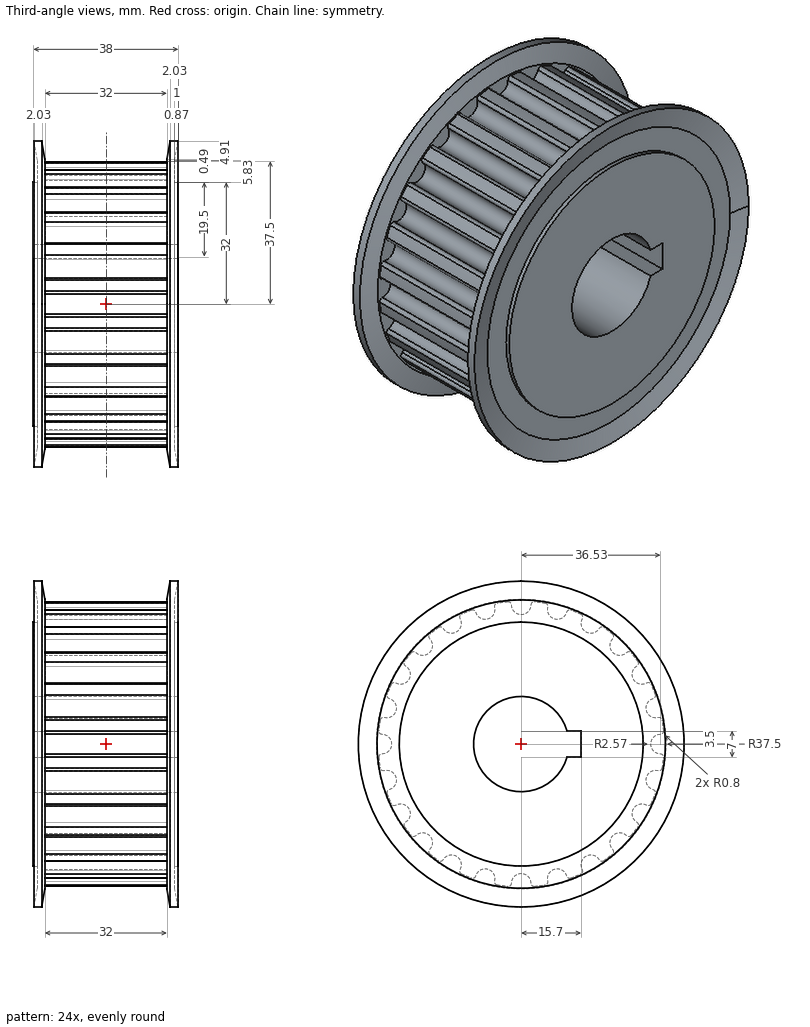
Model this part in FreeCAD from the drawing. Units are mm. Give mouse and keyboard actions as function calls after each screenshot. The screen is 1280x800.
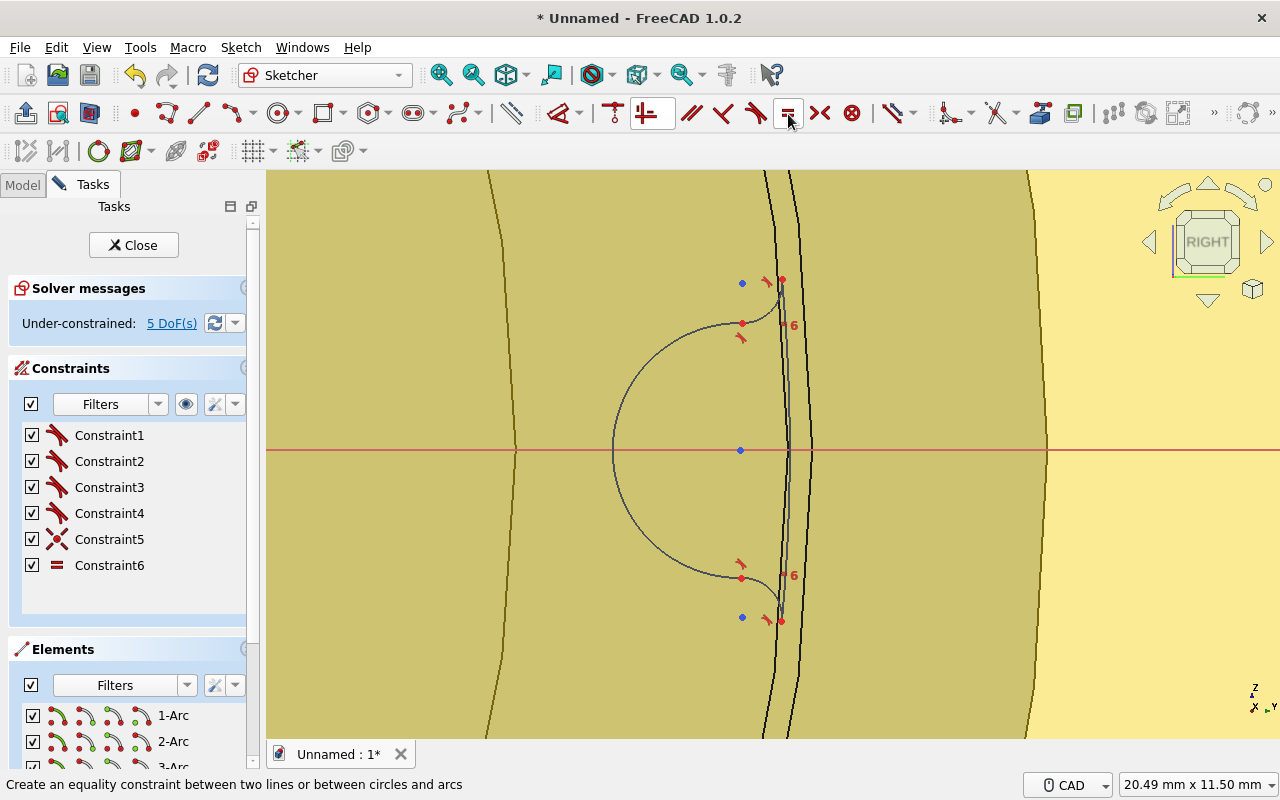
click(740, 451)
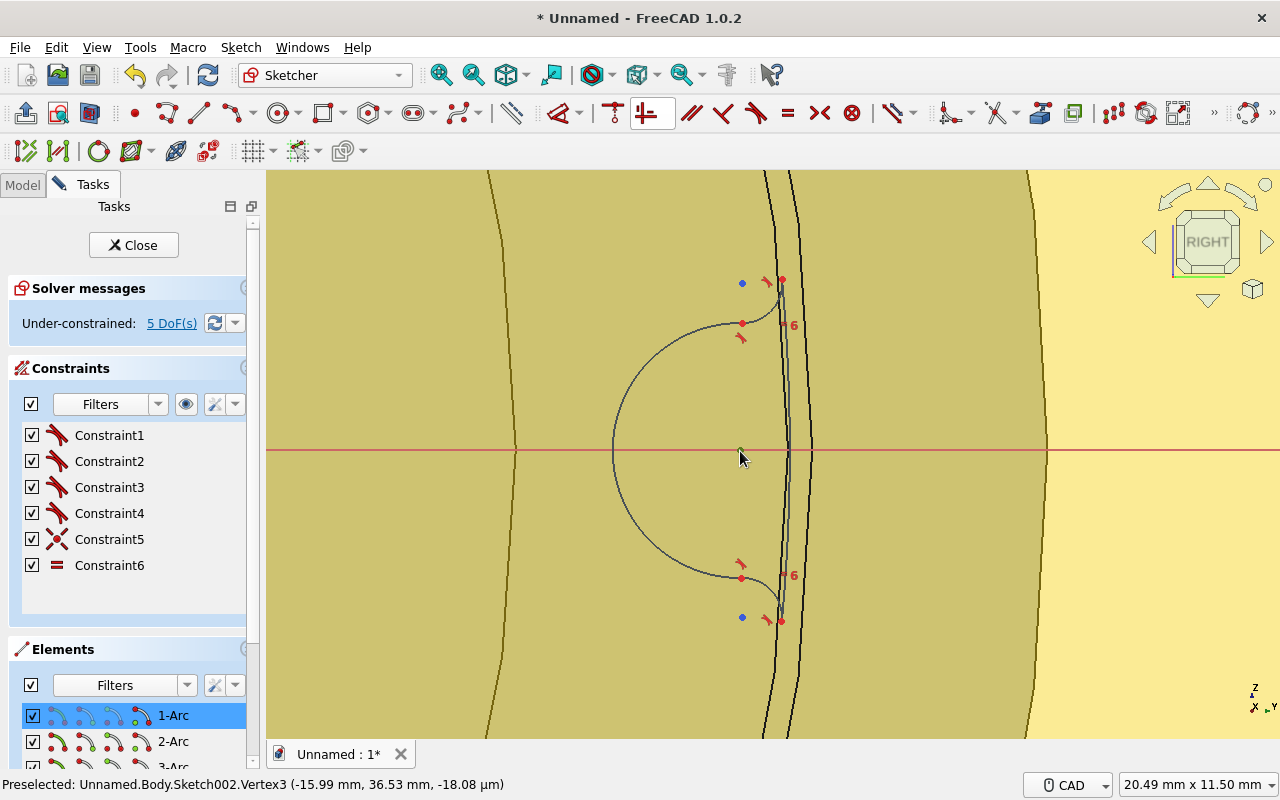
click(353, 450)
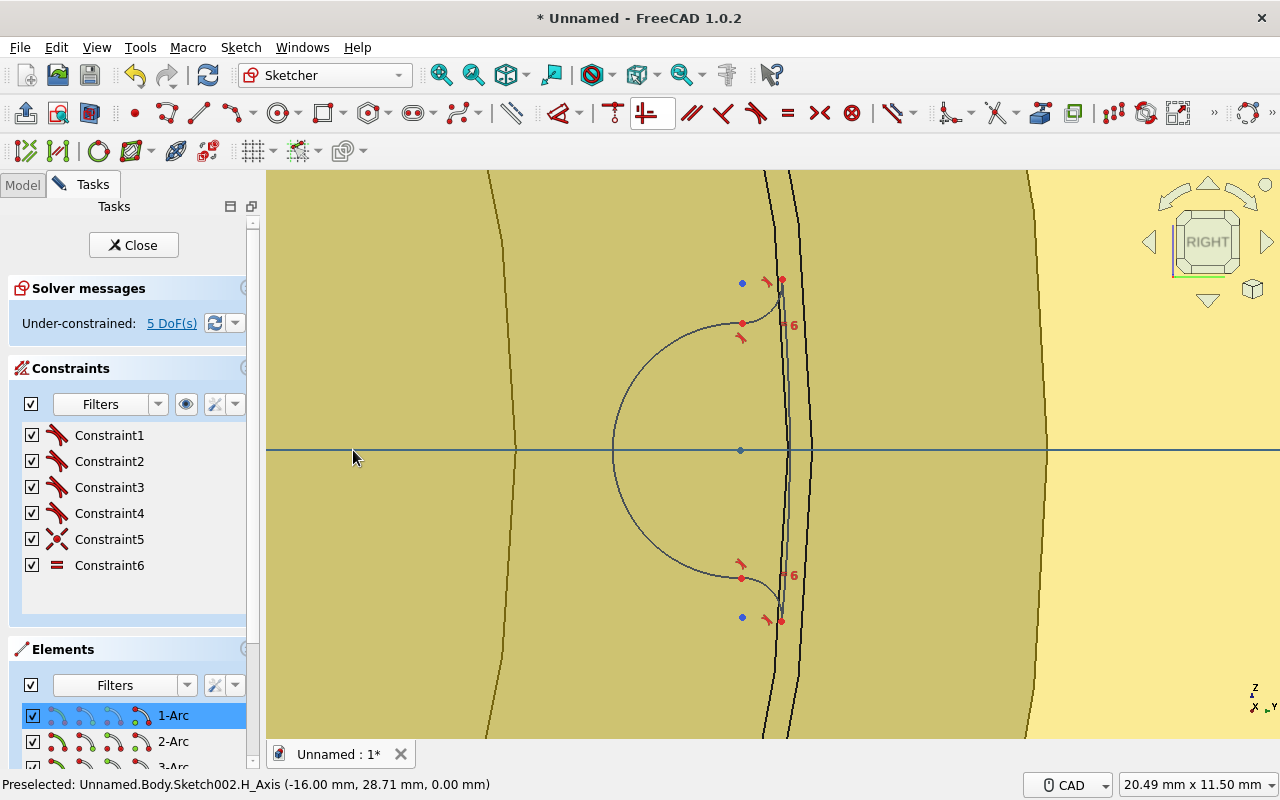
click(614, 114)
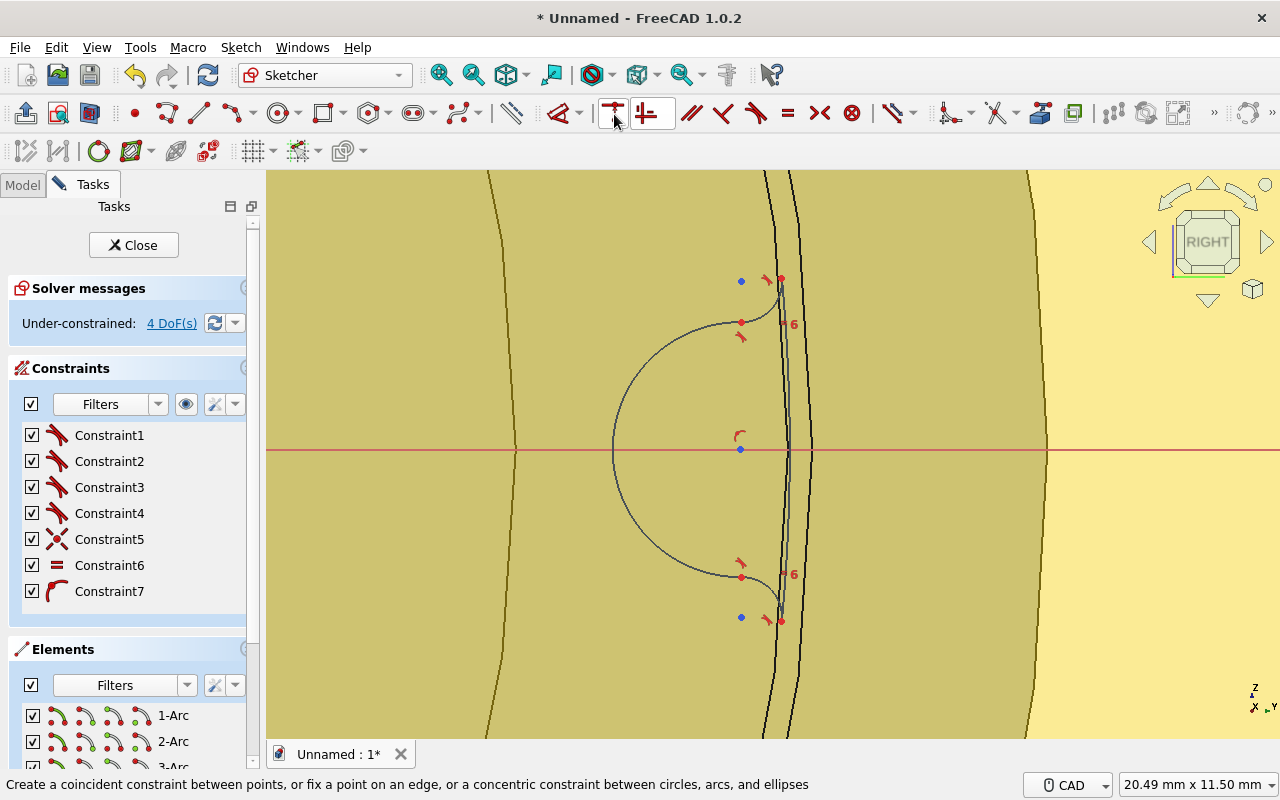
click(558, 114)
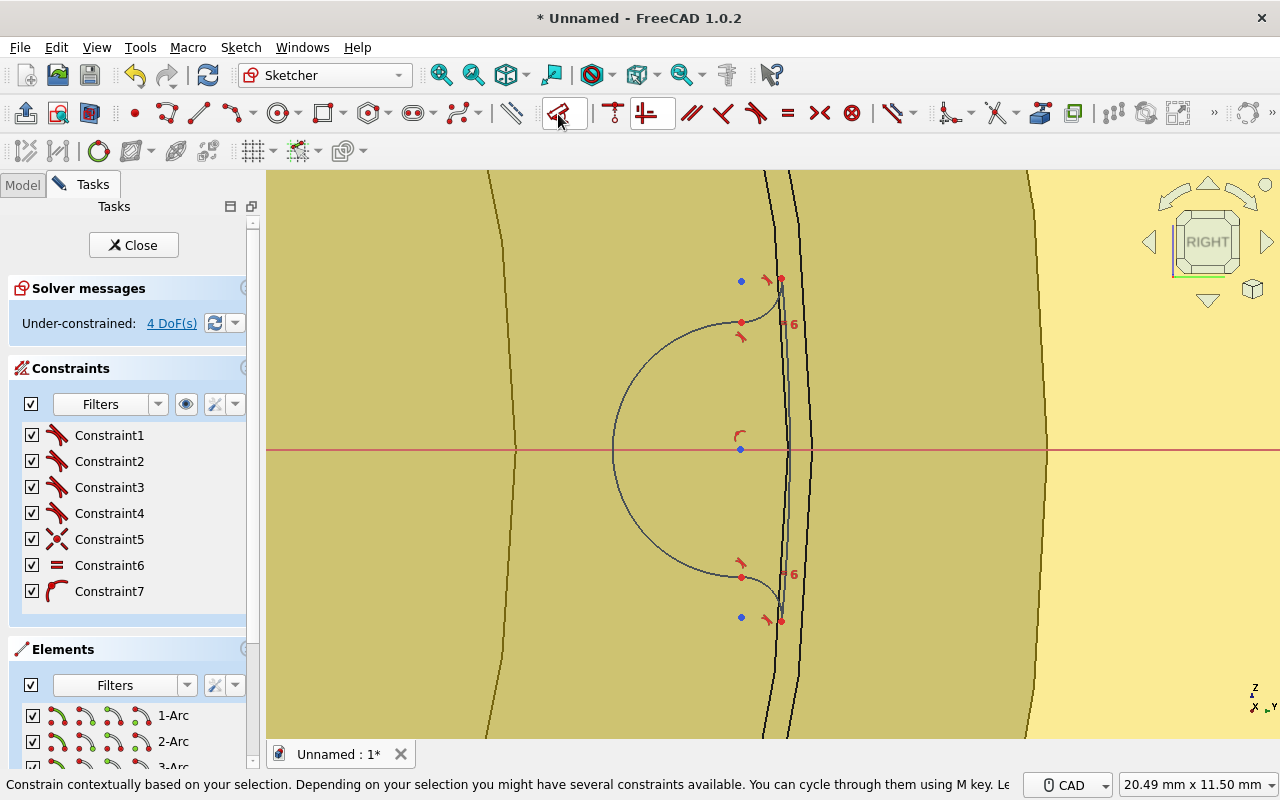
click(637, 374)
click(611, 355)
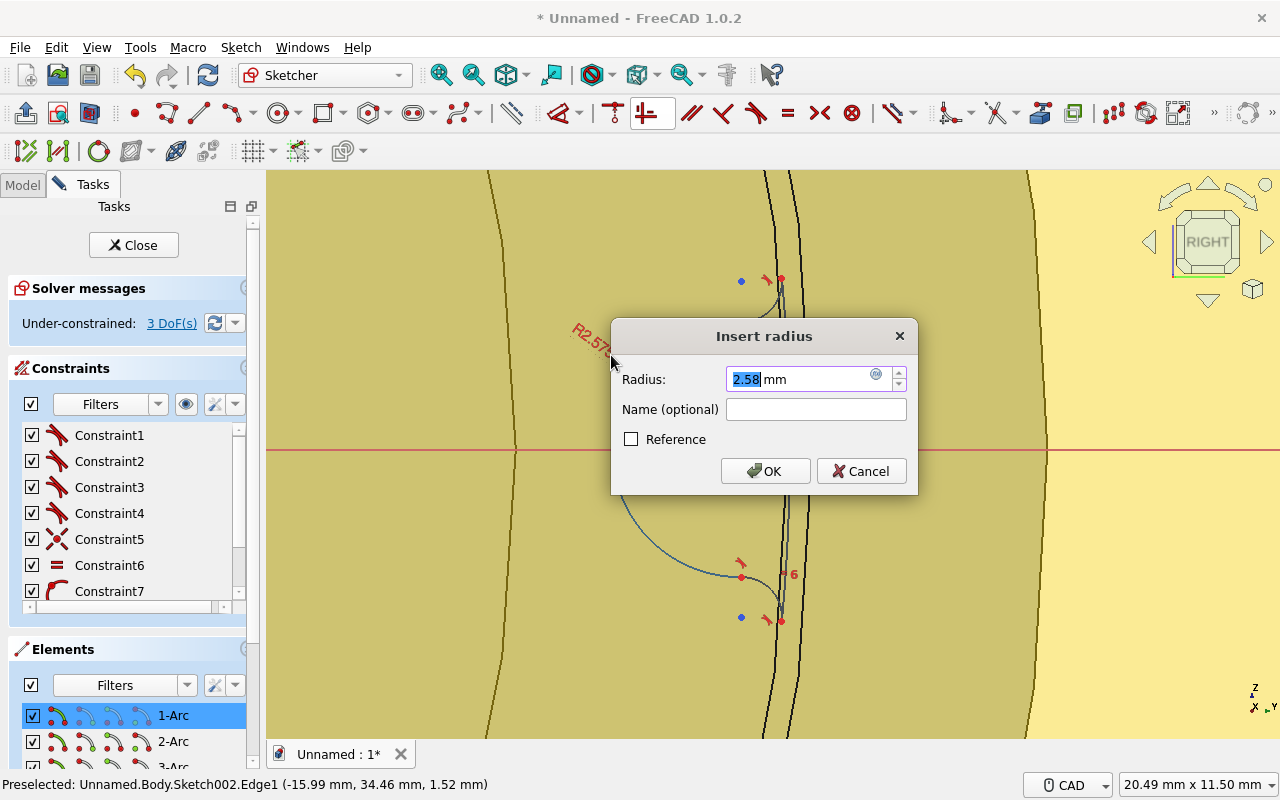
text(2.57)
key(Return)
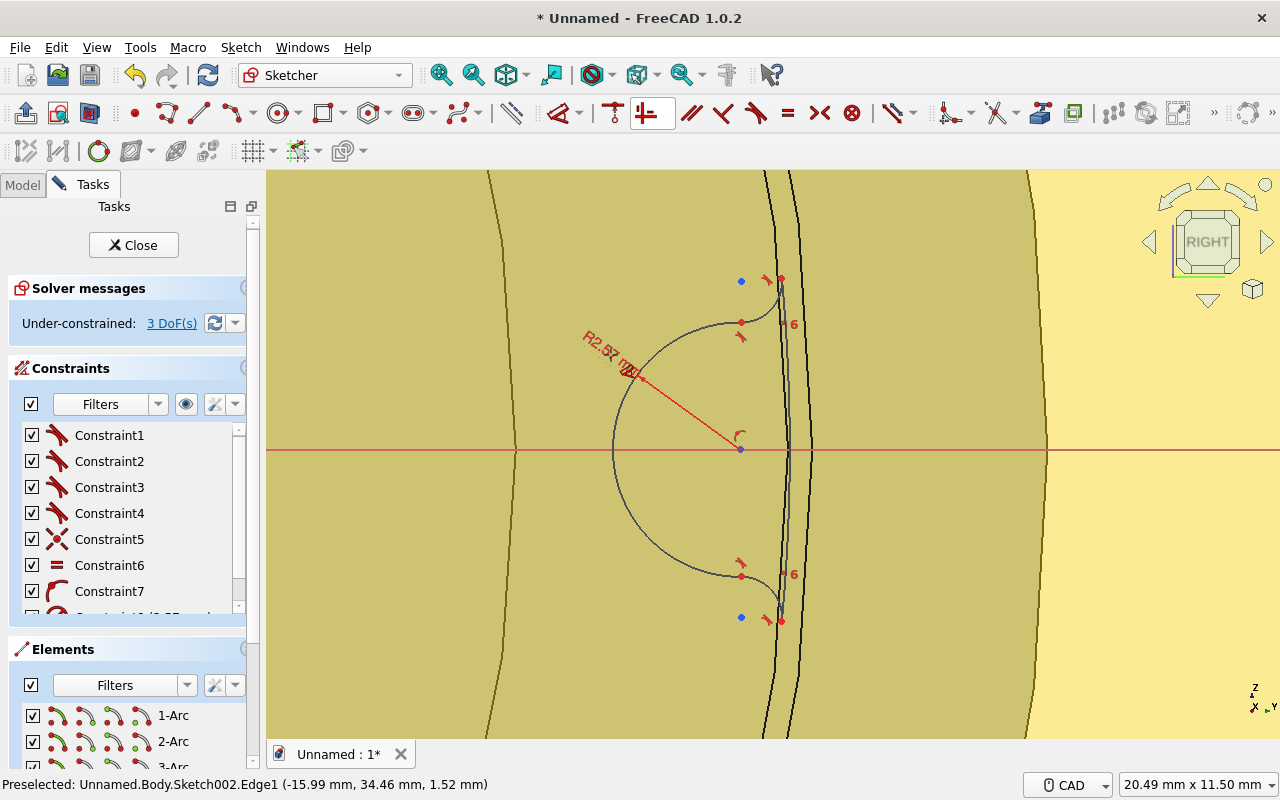
click(761, 582)
click(803, 579)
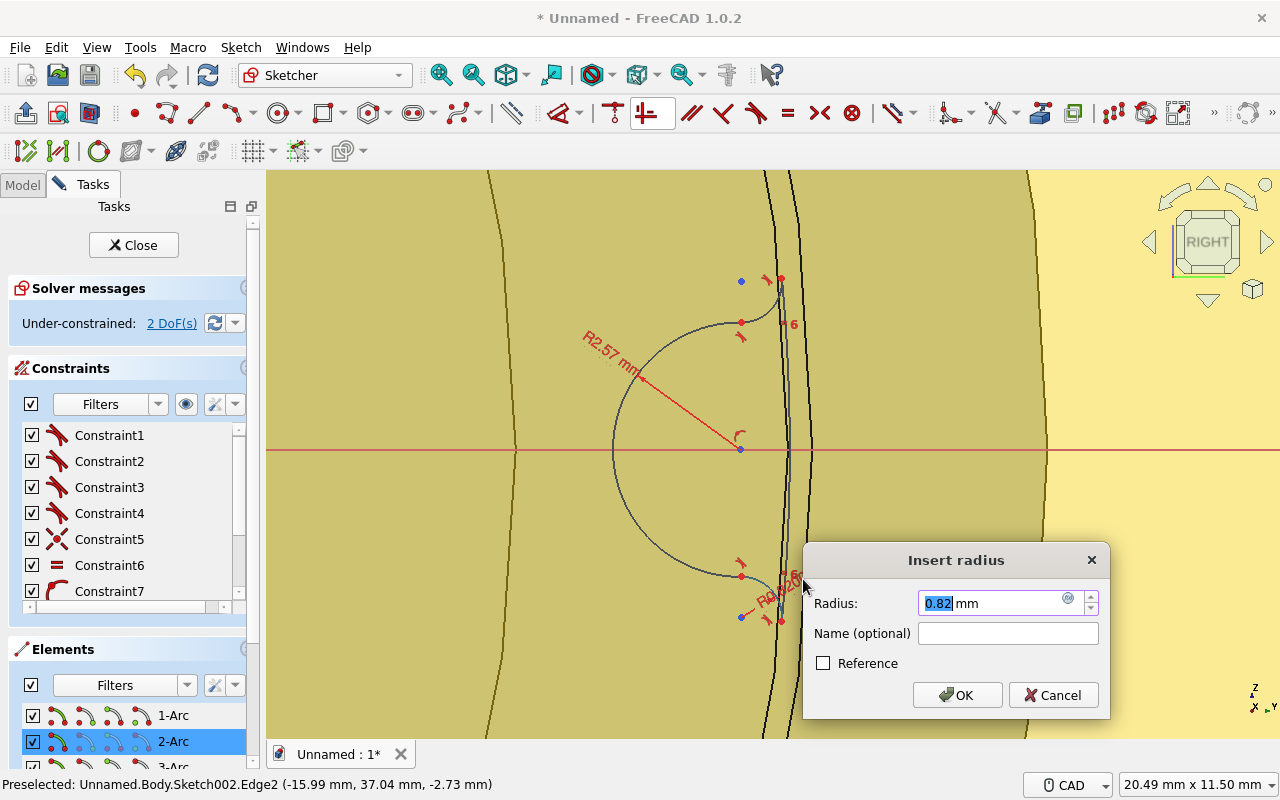
text(0.8)
key(Return)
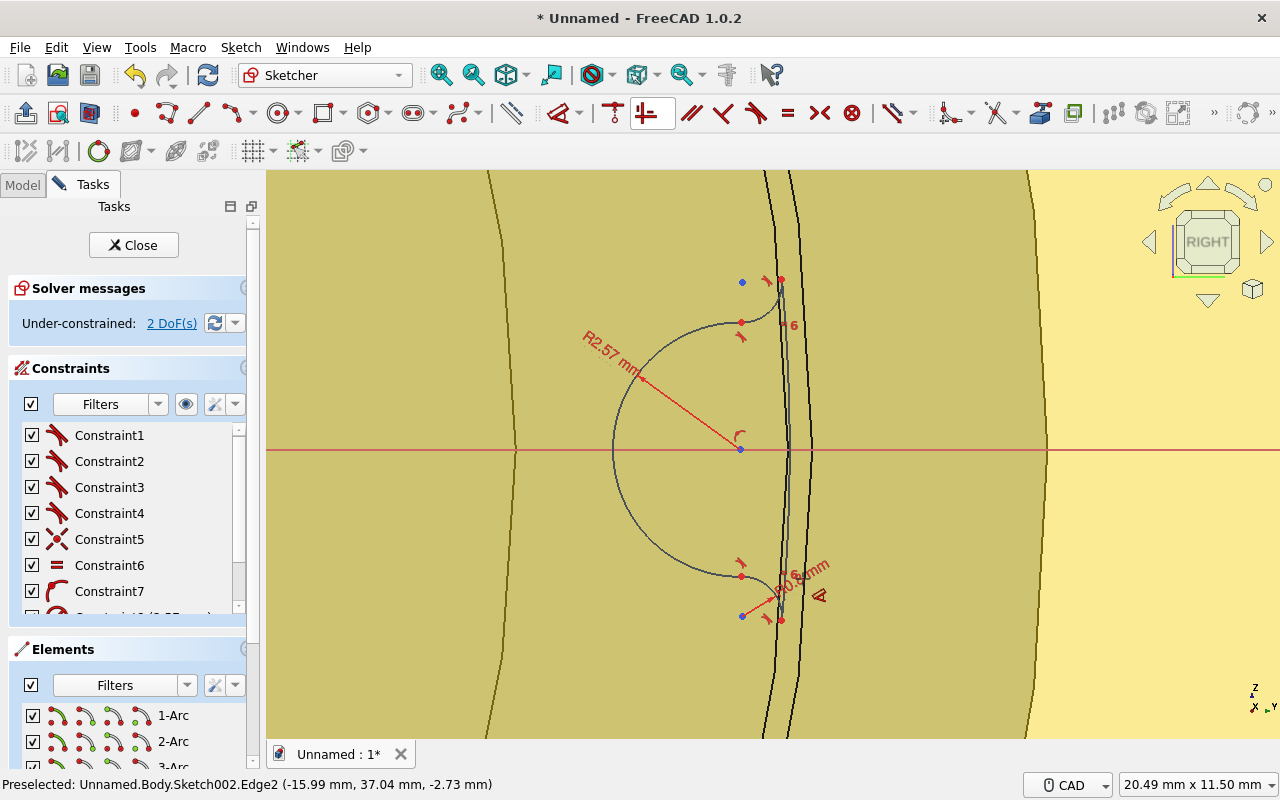
click(788, 518)
click(820, 519)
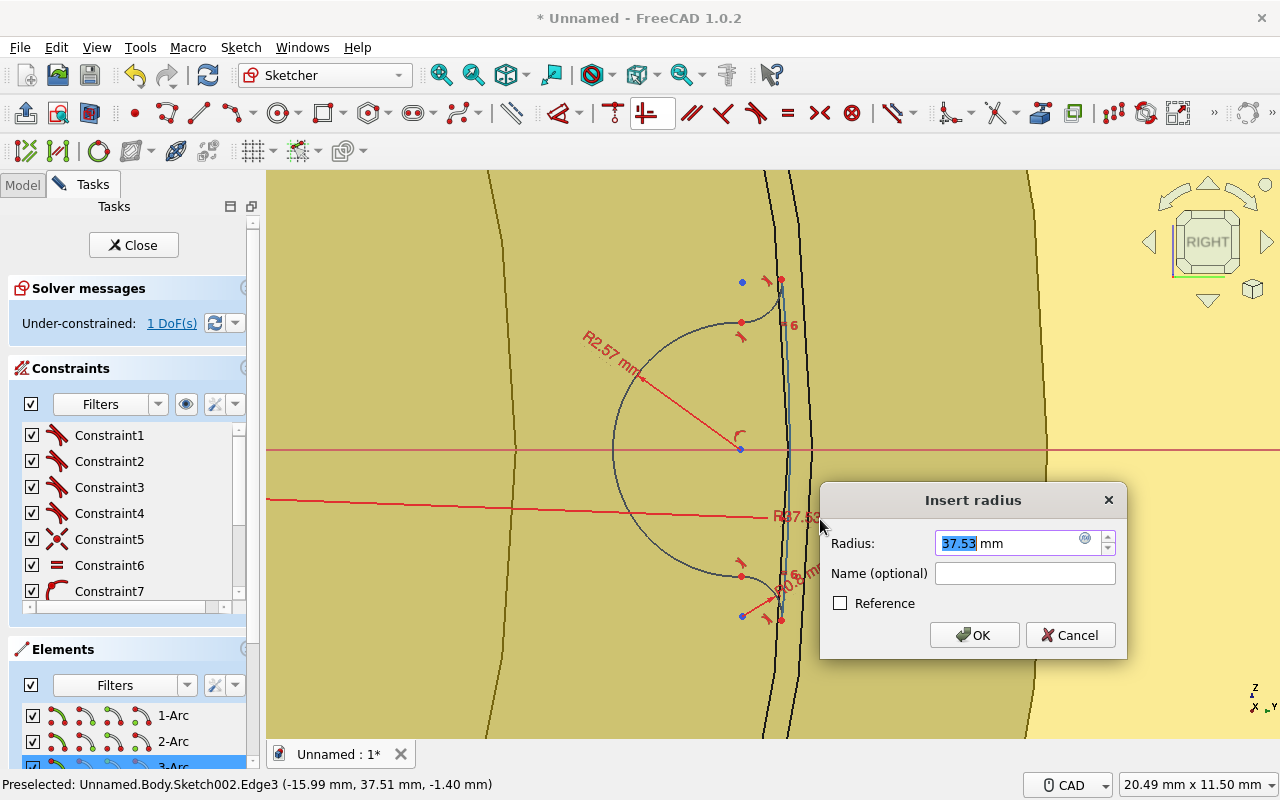
text(37.5)
key(Return)